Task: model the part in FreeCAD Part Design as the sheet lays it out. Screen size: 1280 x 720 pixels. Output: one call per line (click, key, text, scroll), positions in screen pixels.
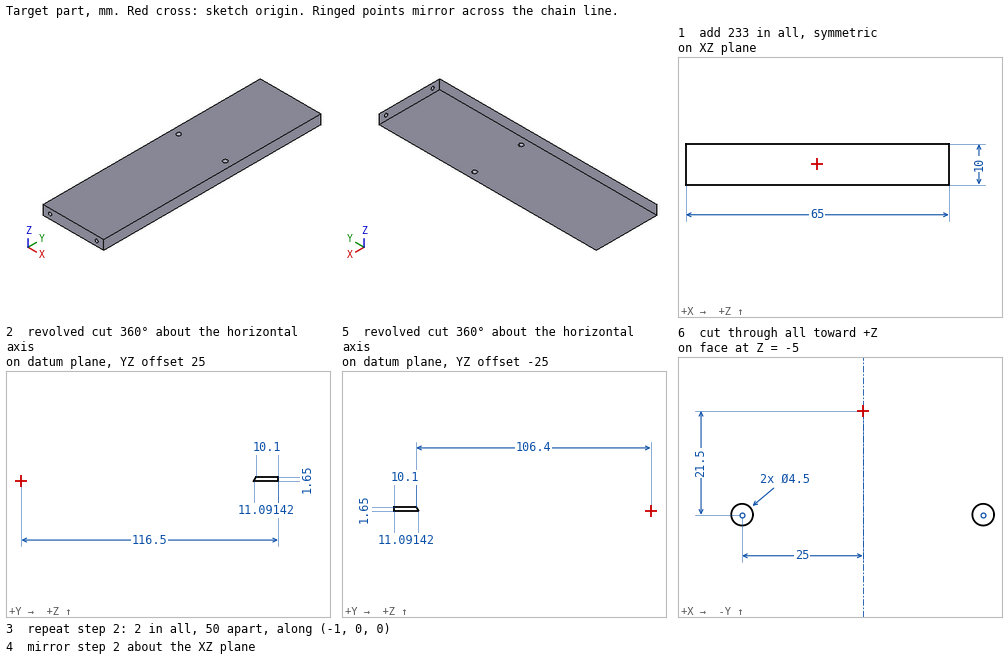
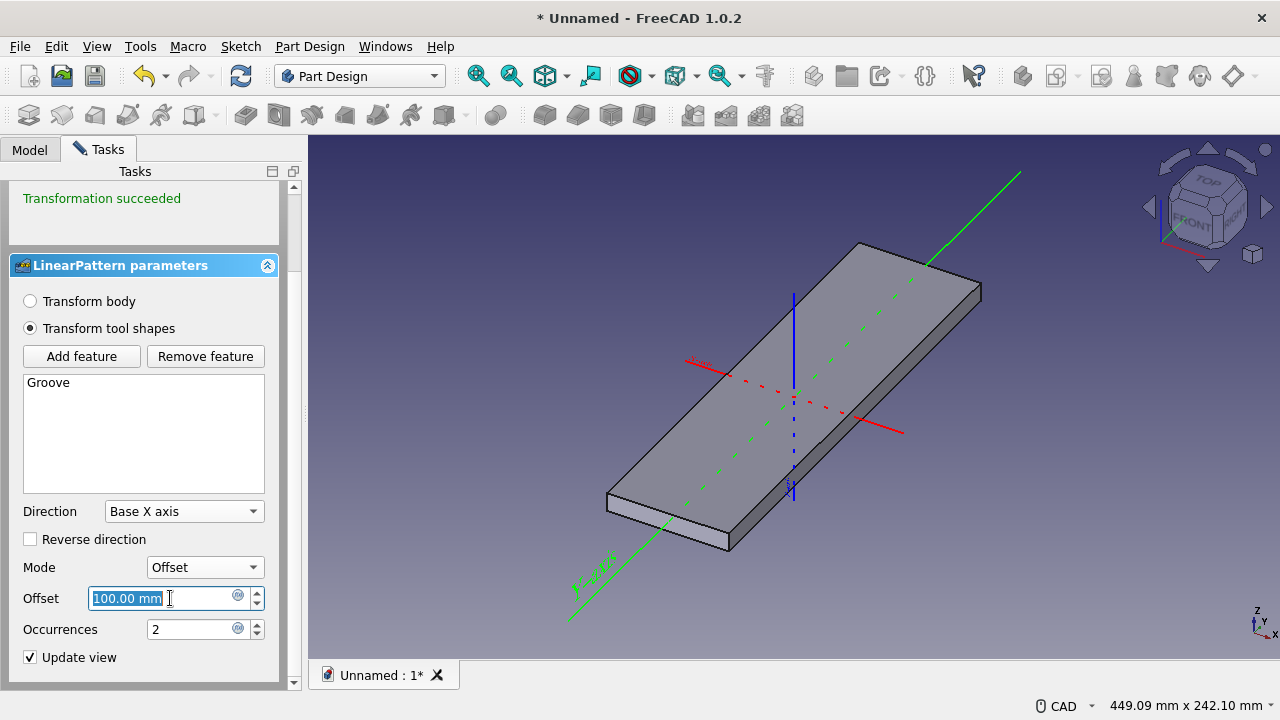
text(50)
key(Tab)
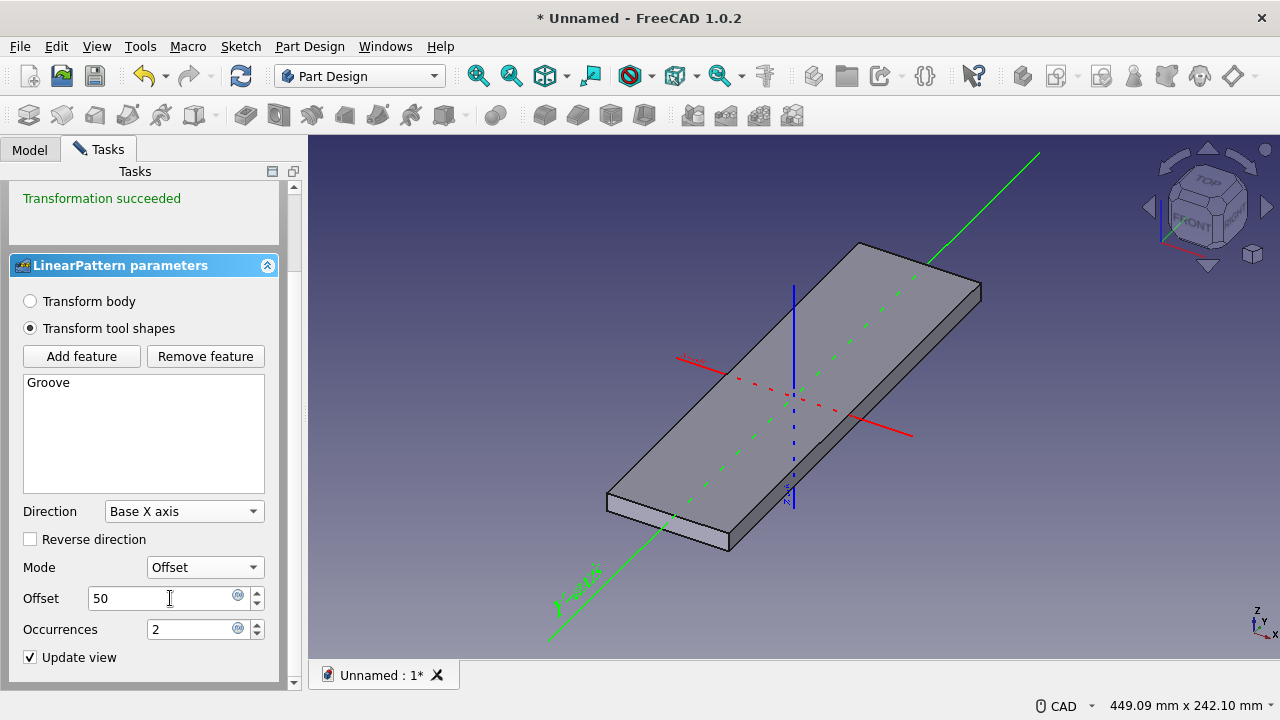
triple_click(199, 630)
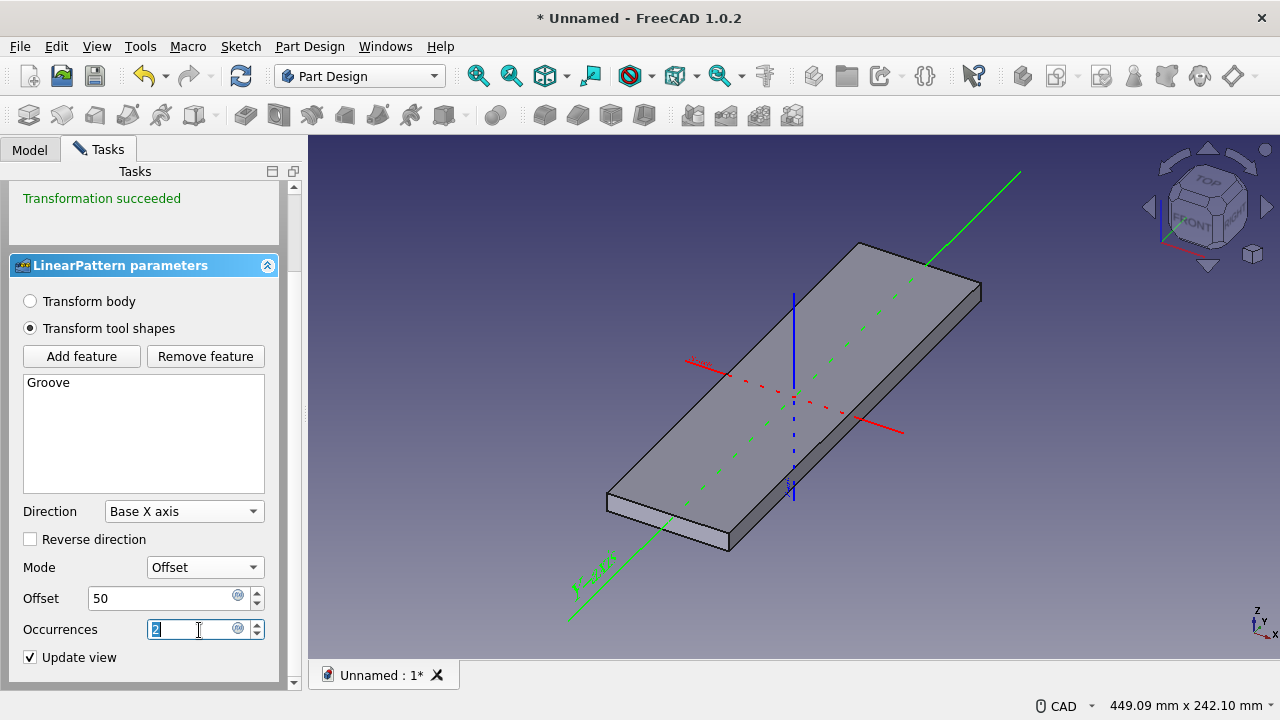
text(2)
key(Tab)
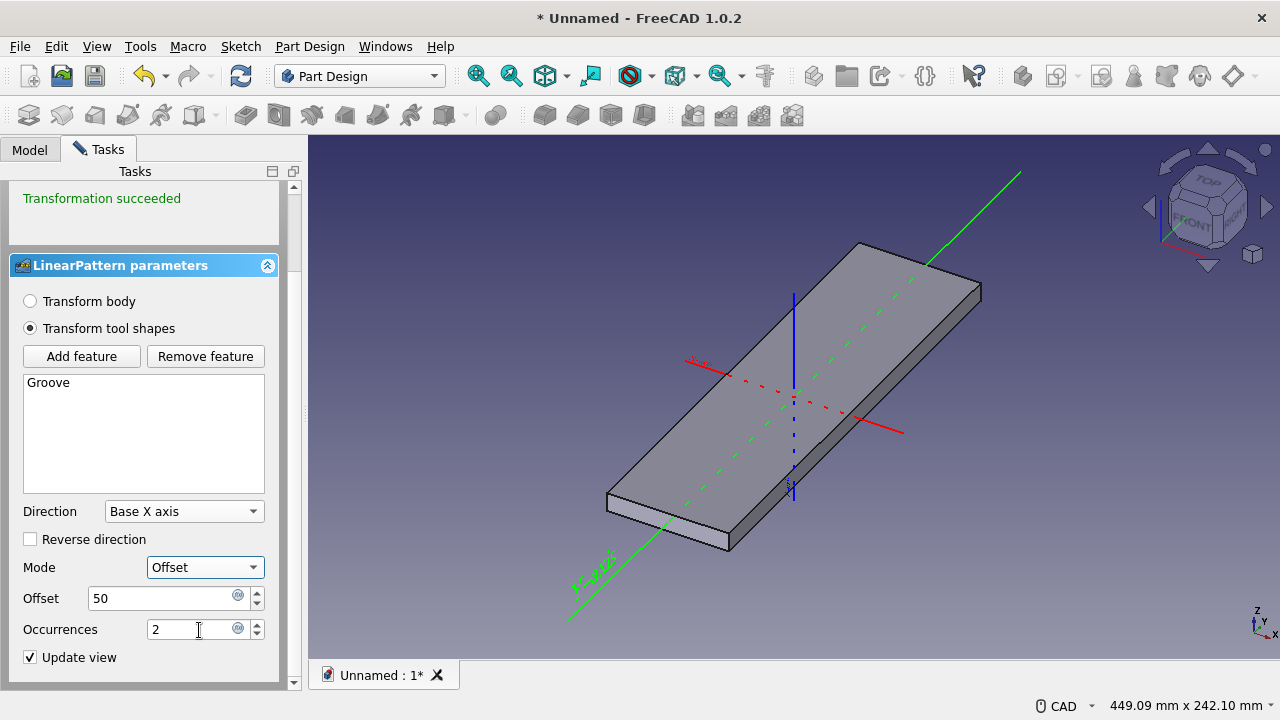
click(31, 539)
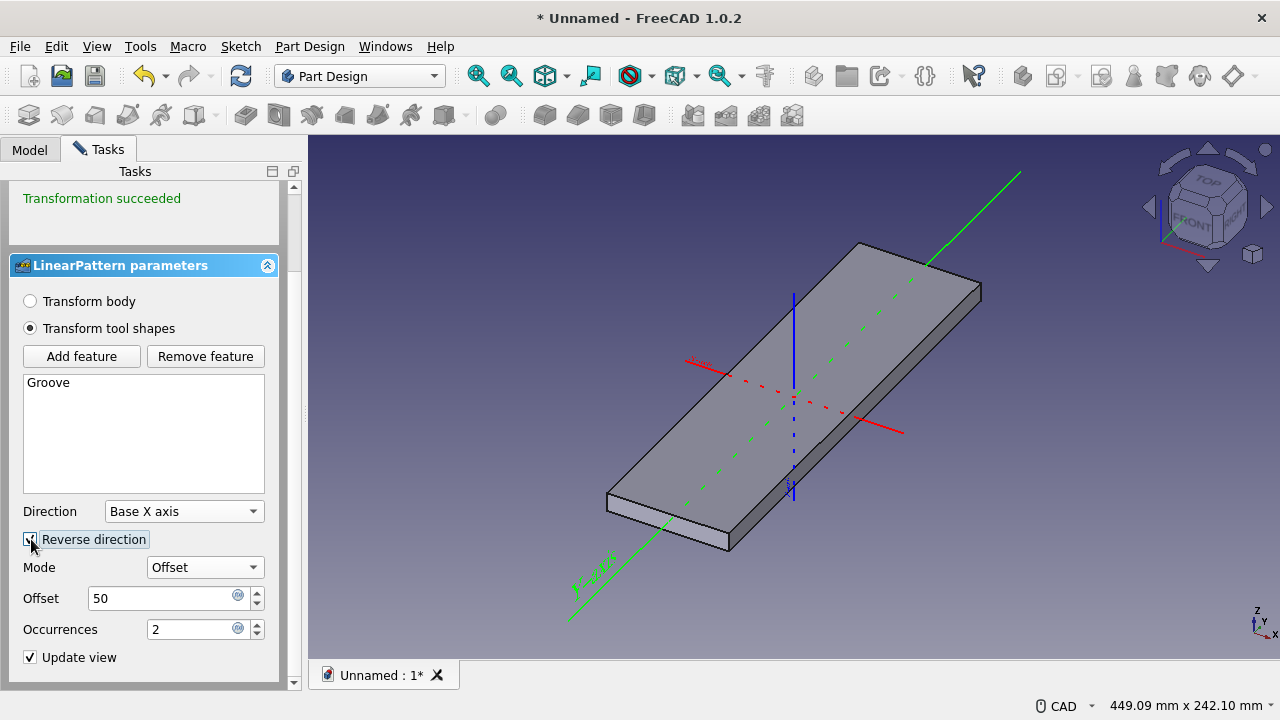
scroll(294, 436, up, 3)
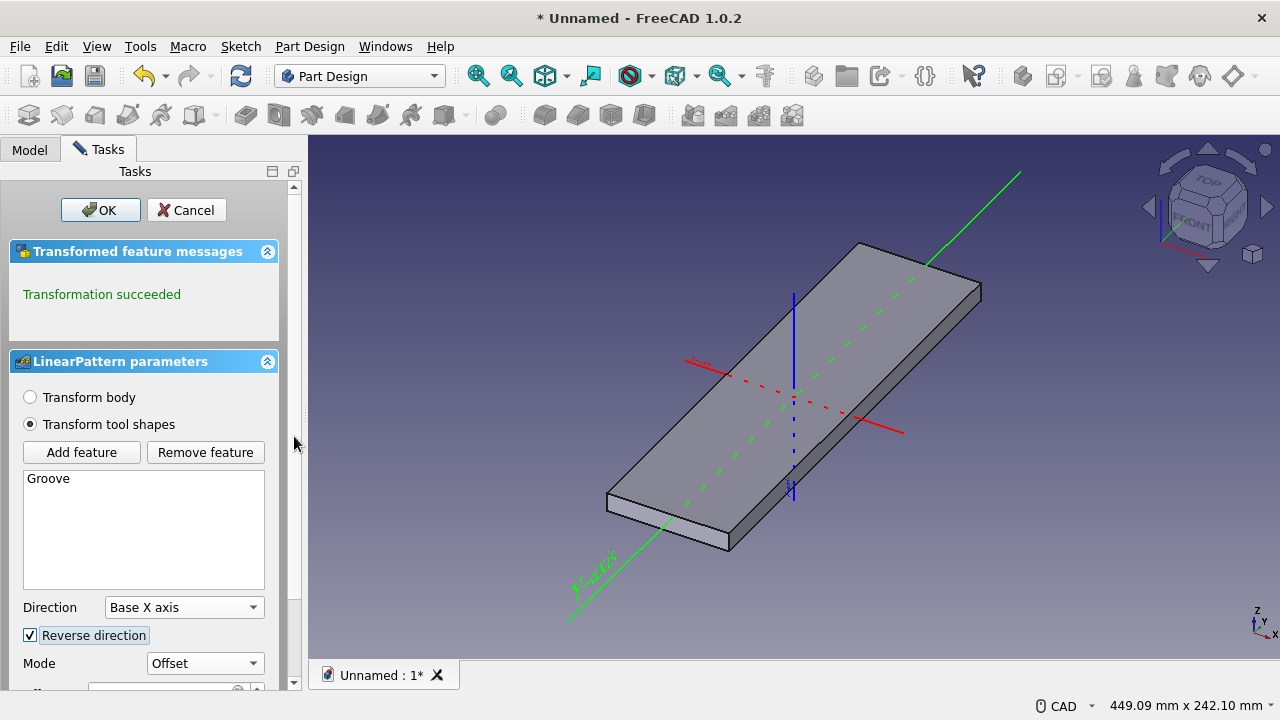
click(101, 210)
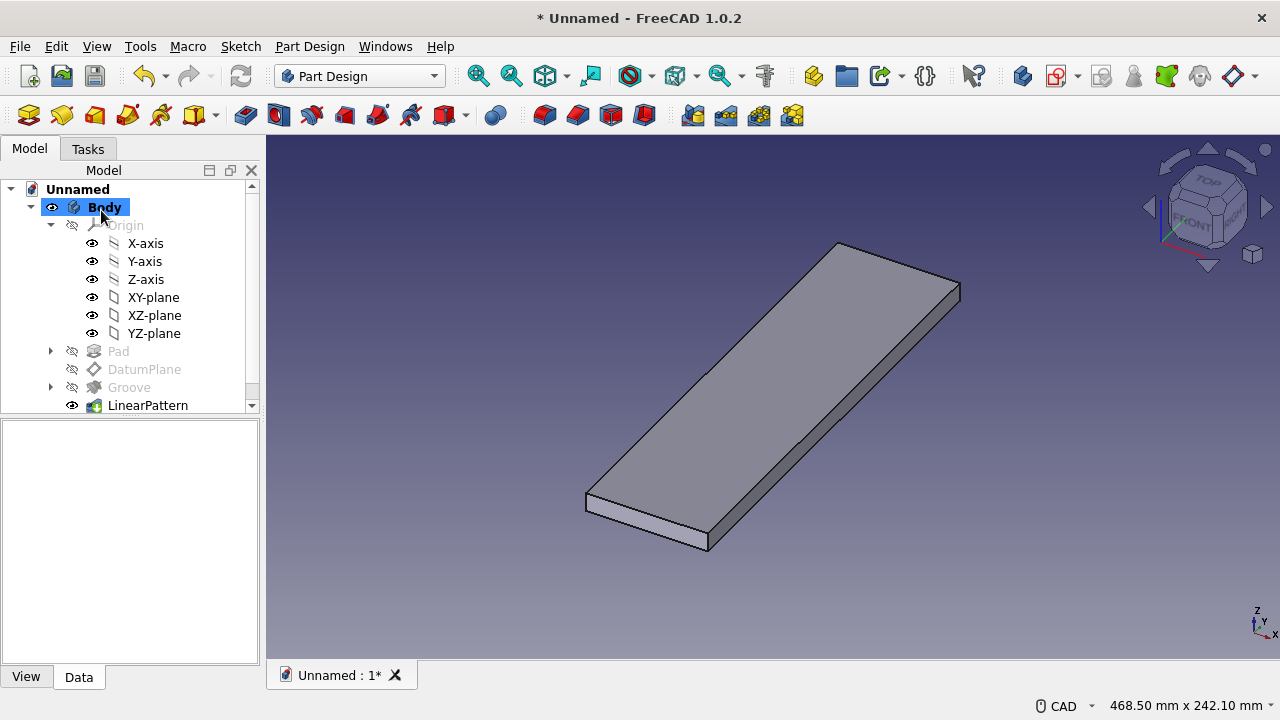
click(117, 387)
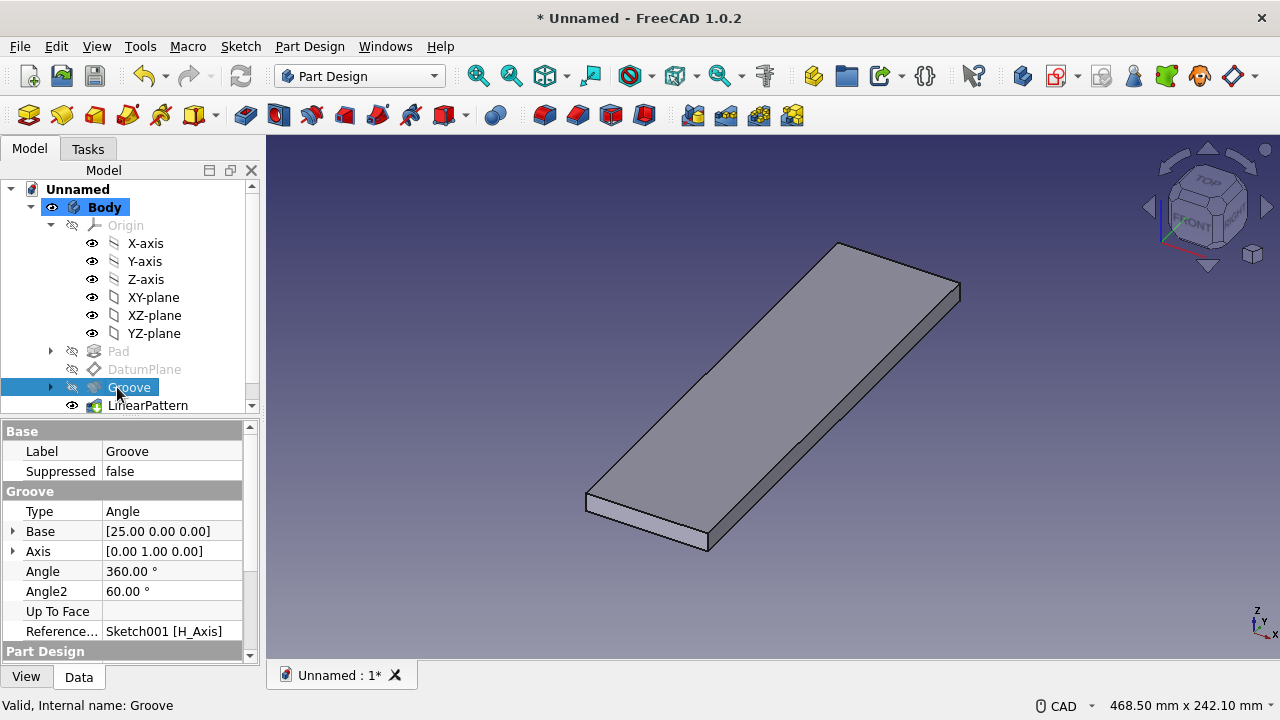
click(693, 116)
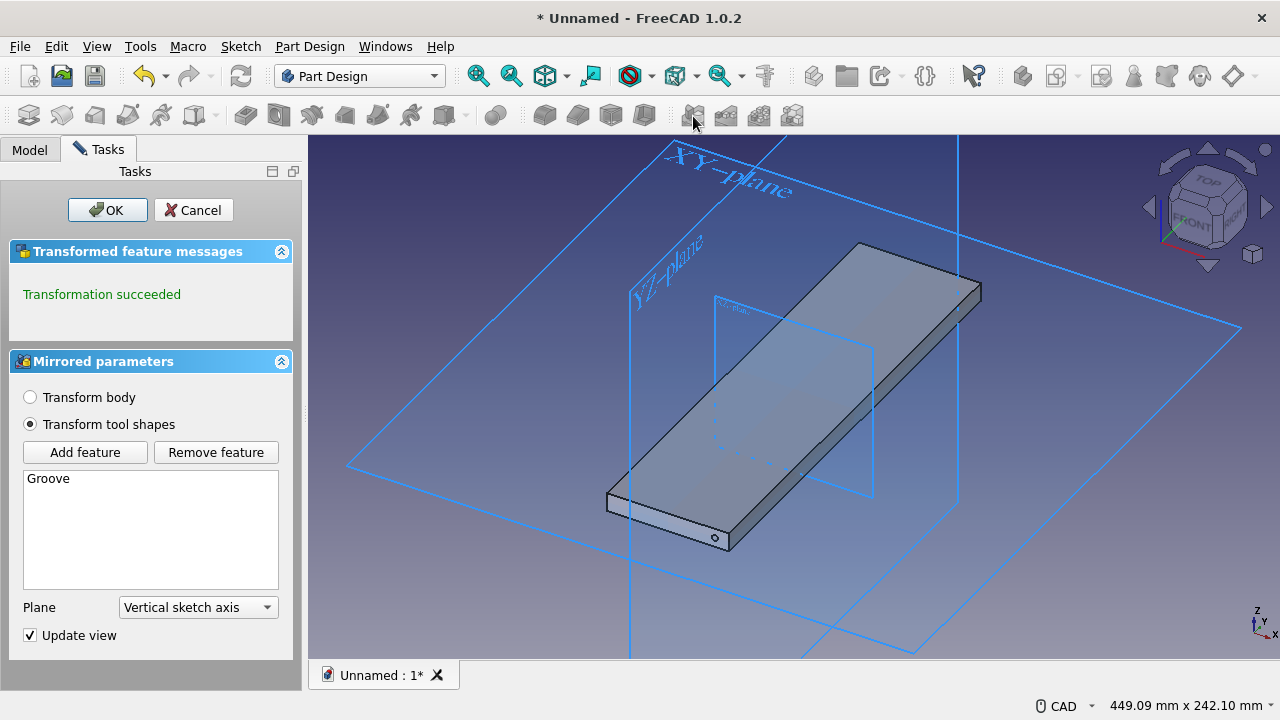
click(199, 608)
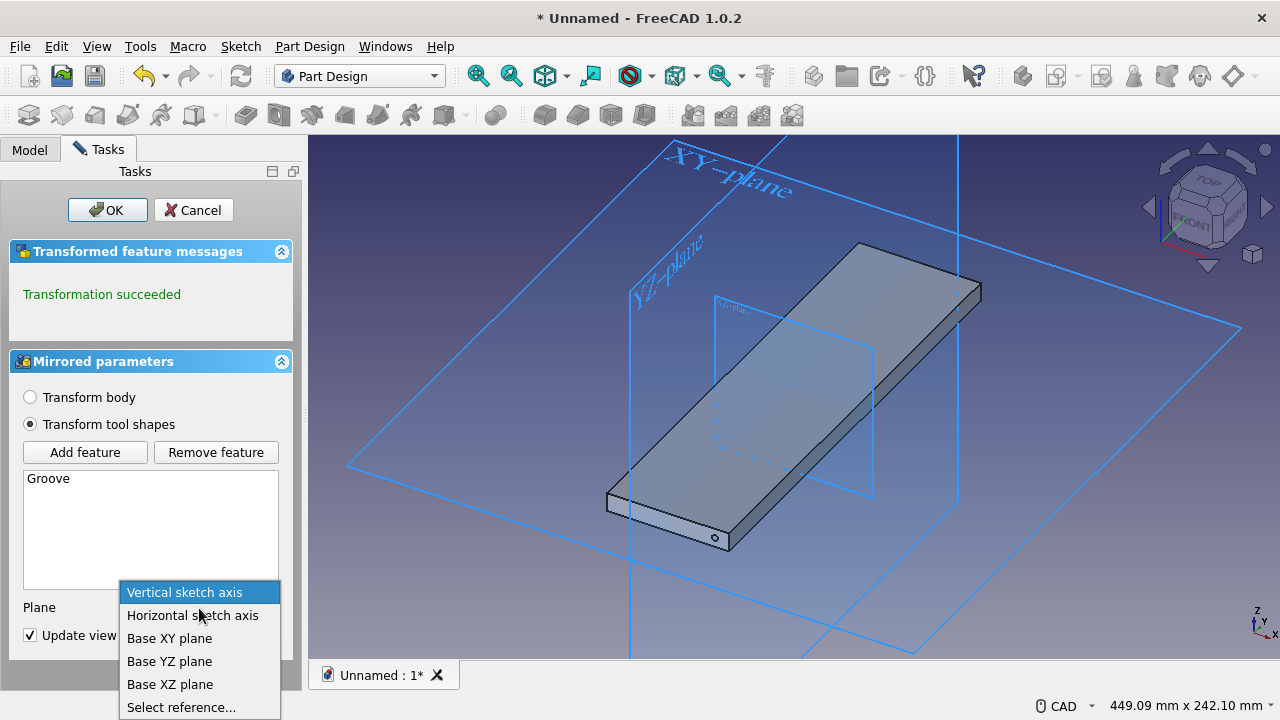
click(198, 684)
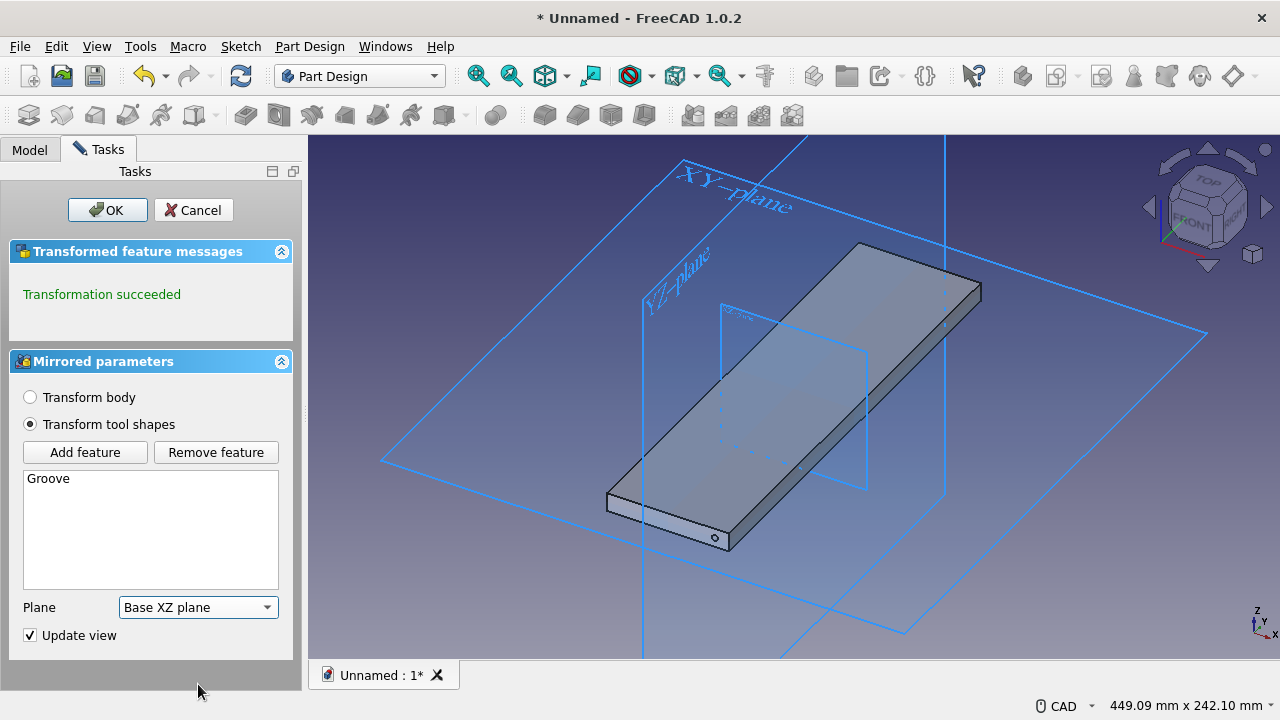
click(108, 210)